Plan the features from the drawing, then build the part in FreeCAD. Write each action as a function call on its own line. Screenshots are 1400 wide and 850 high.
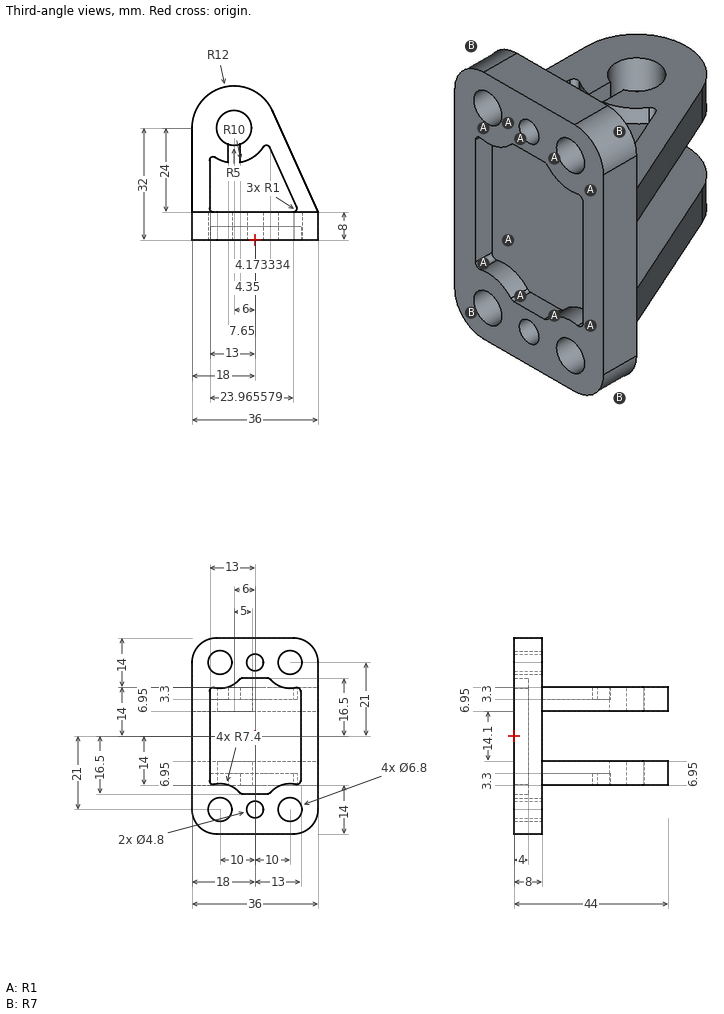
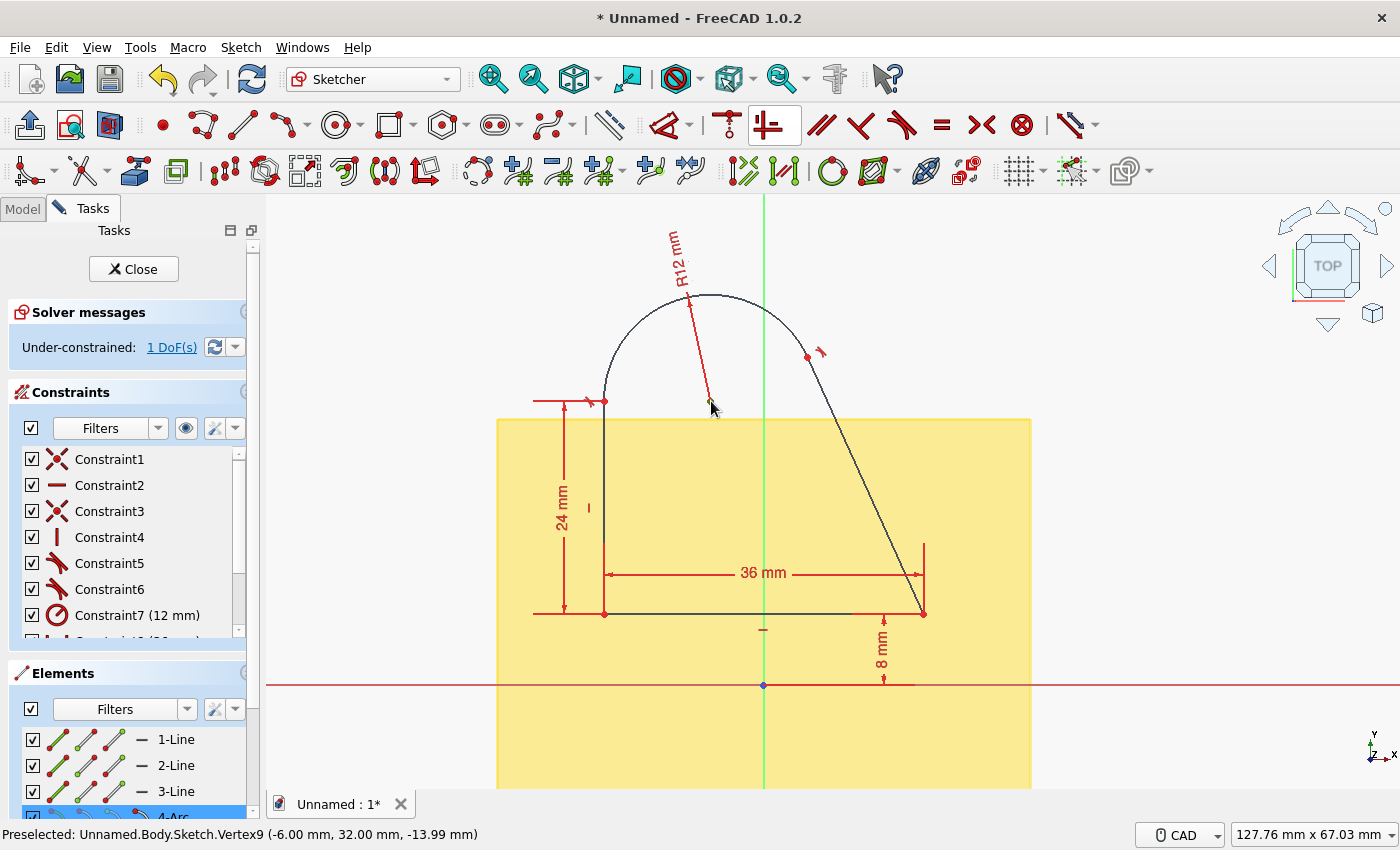
key(l)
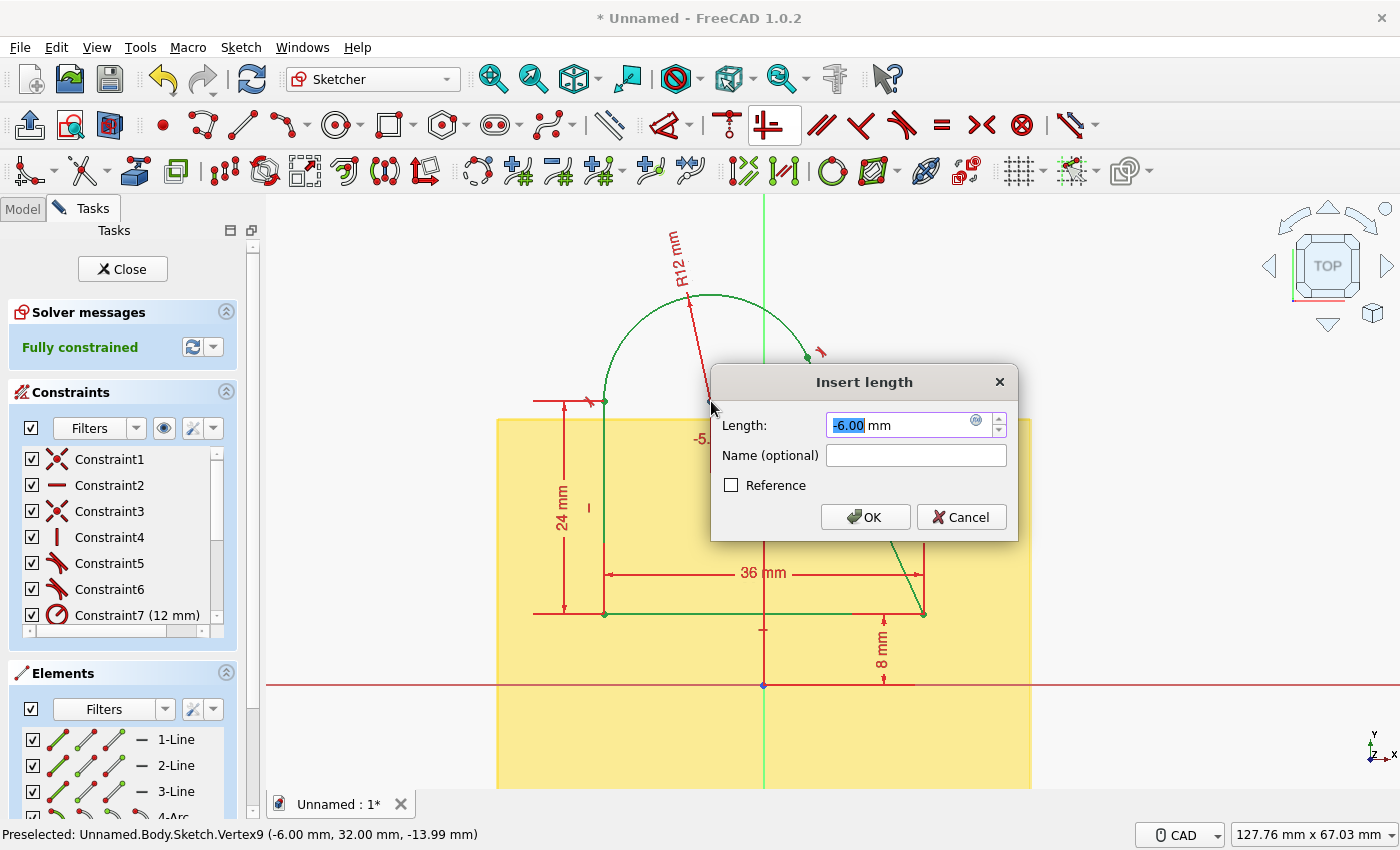
text(-6)
key(Return)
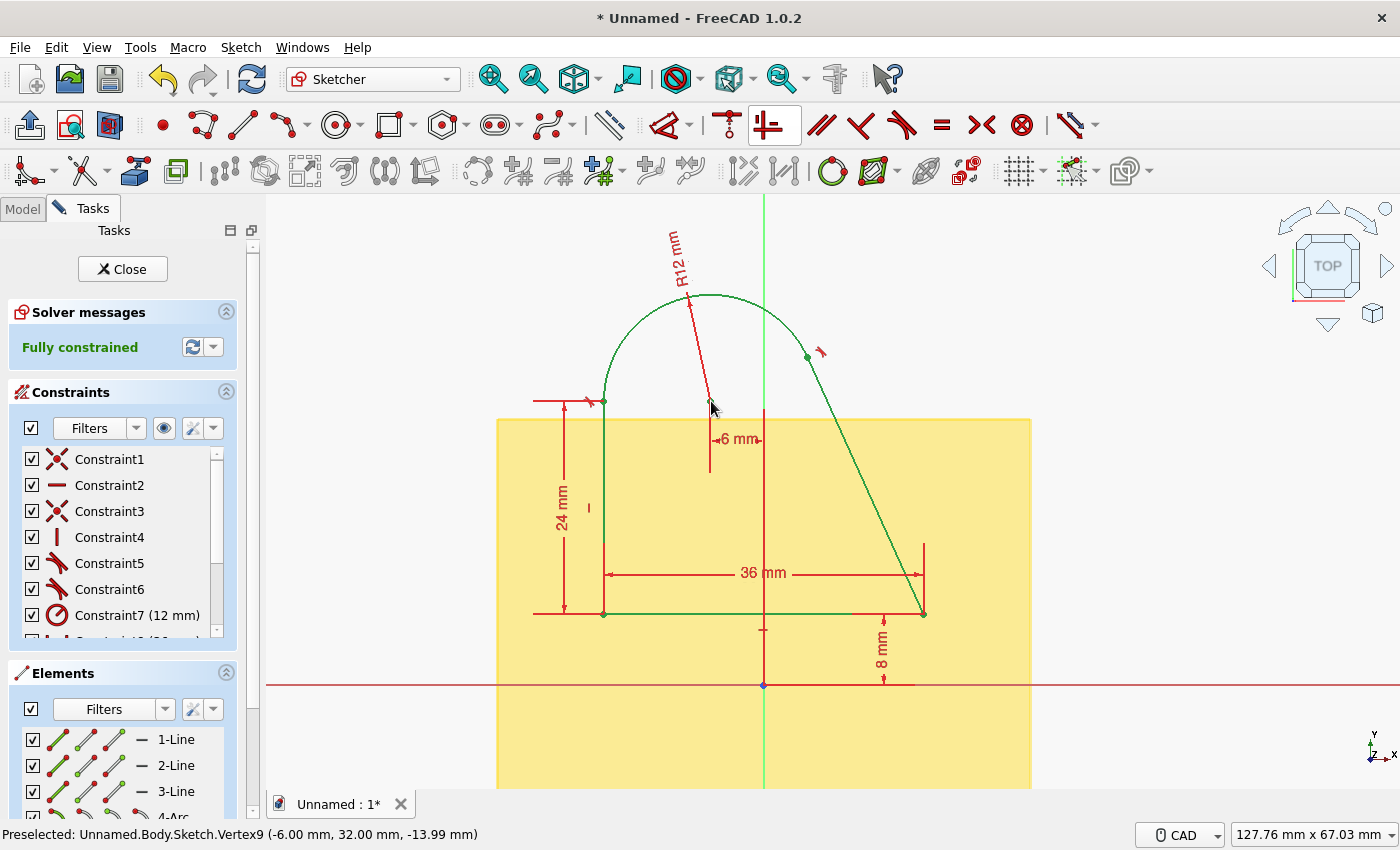
click(123, 269)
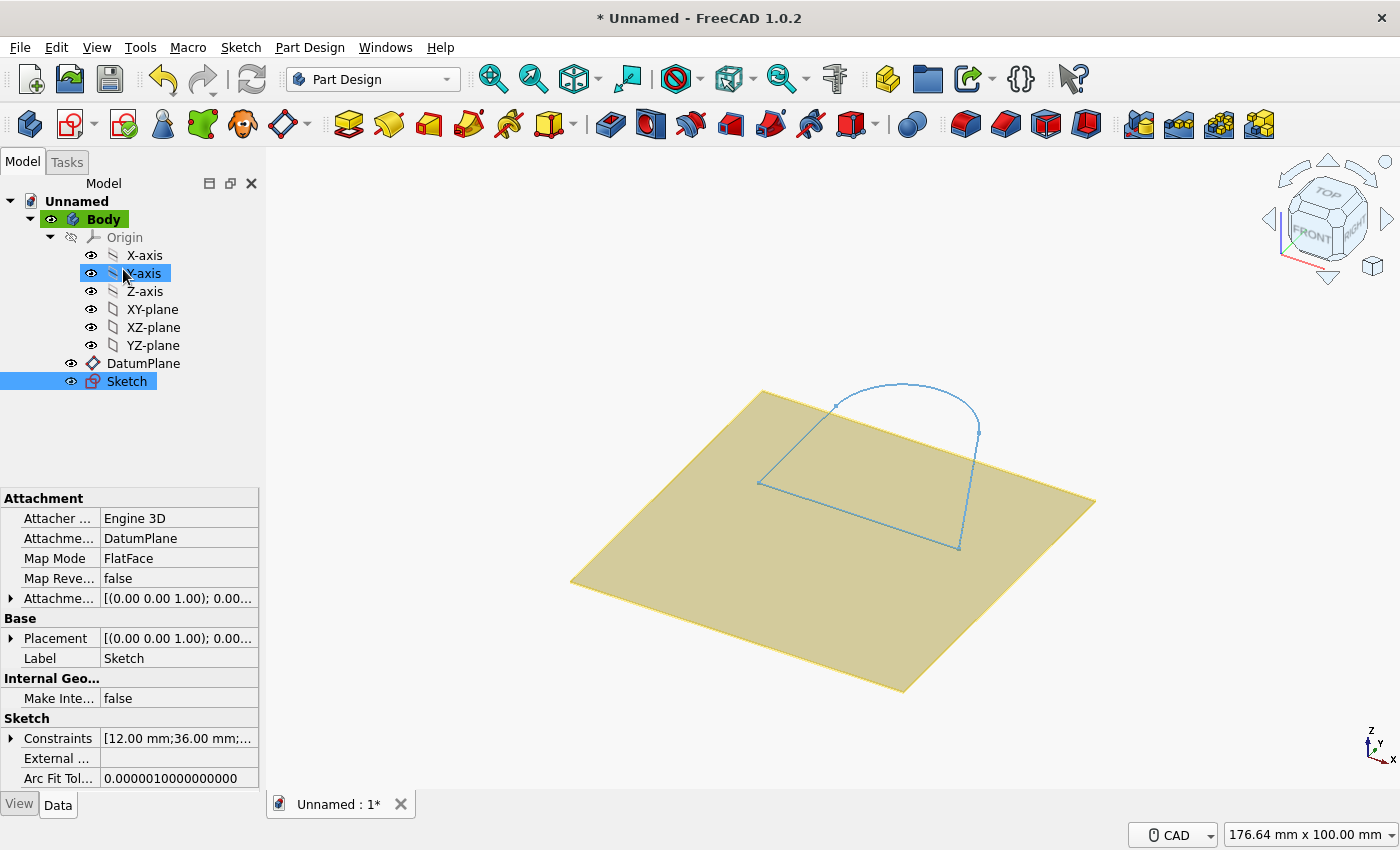
click(350, 124)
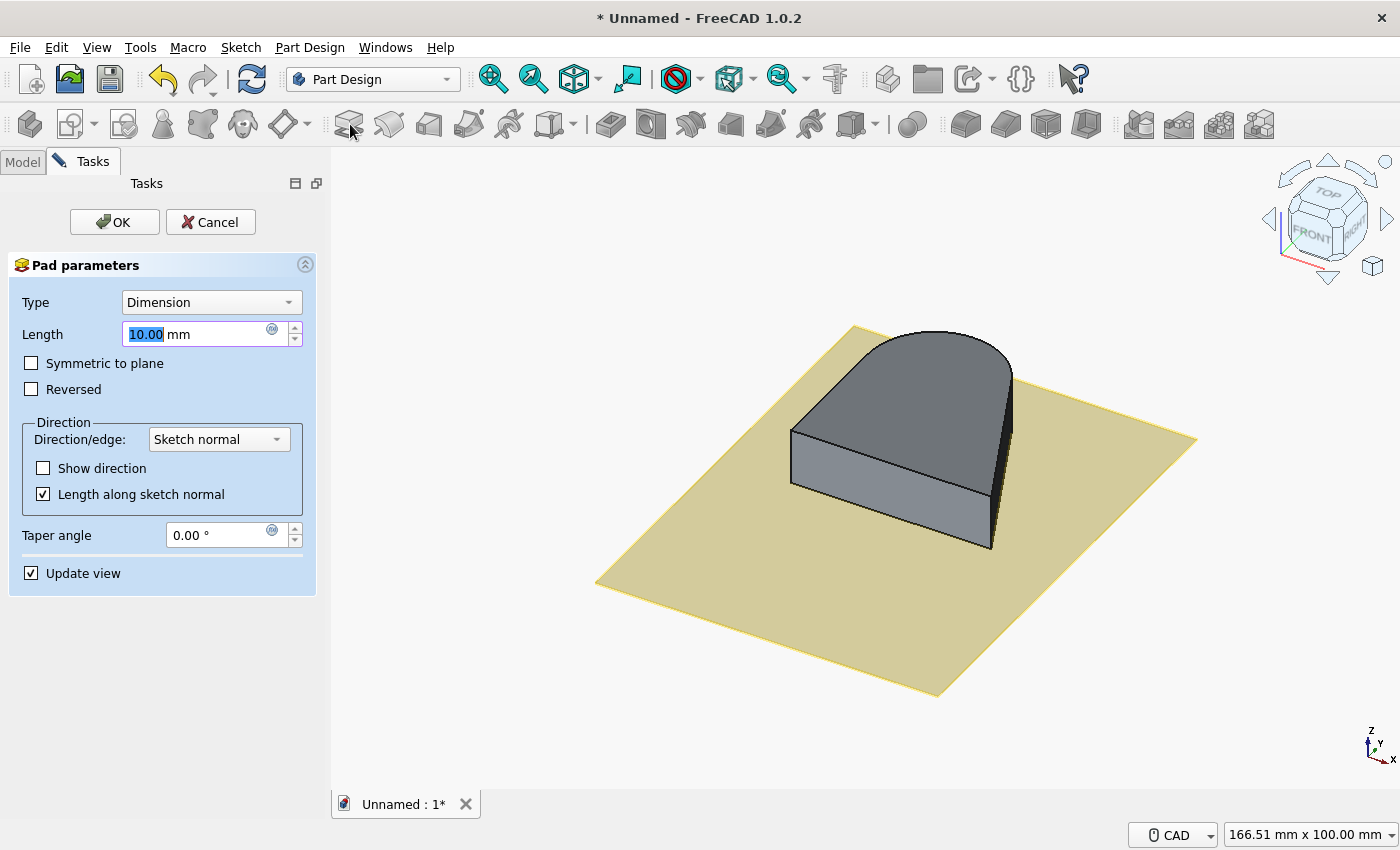
text(6.95)
key(Tab)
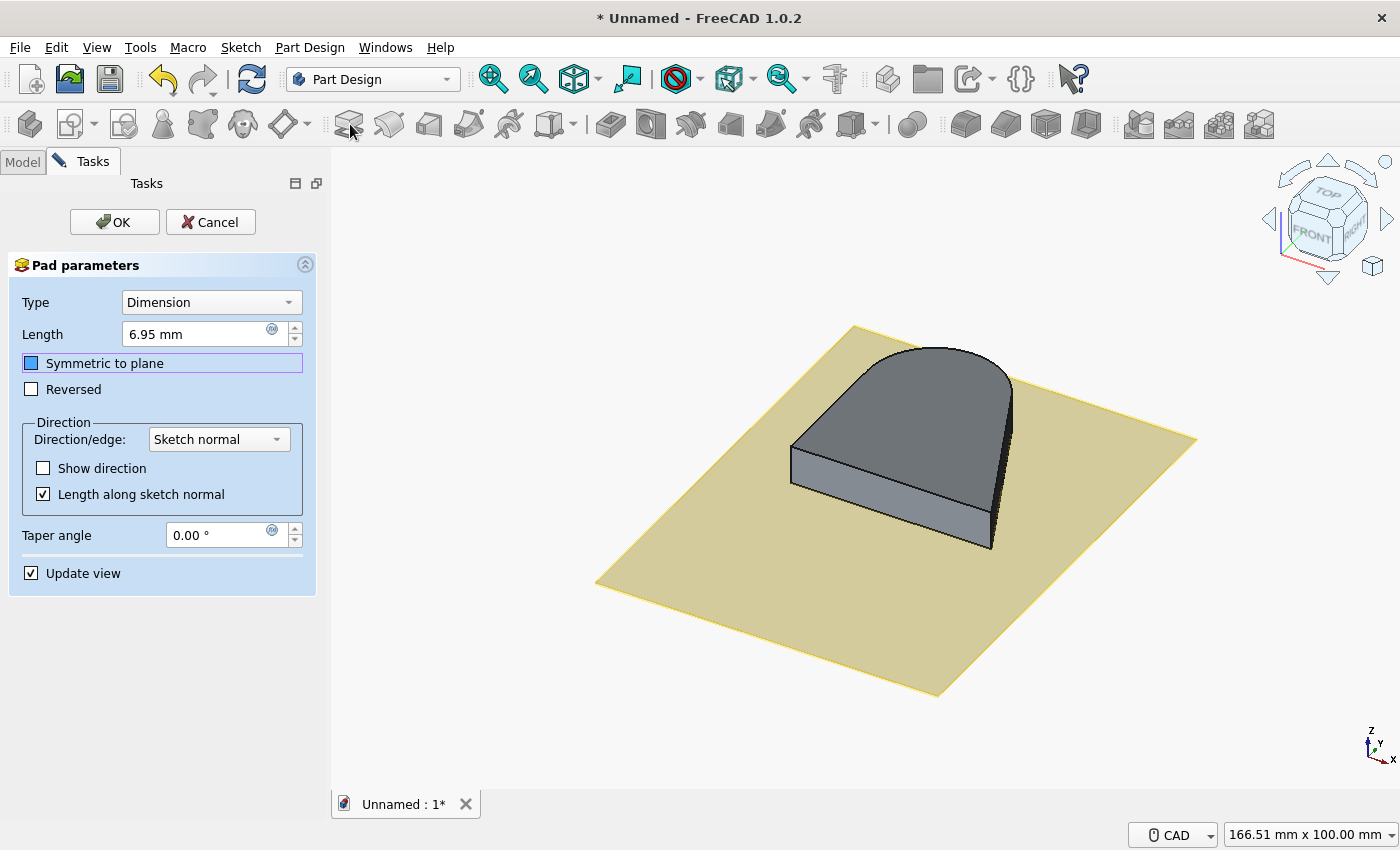
click(115, 222)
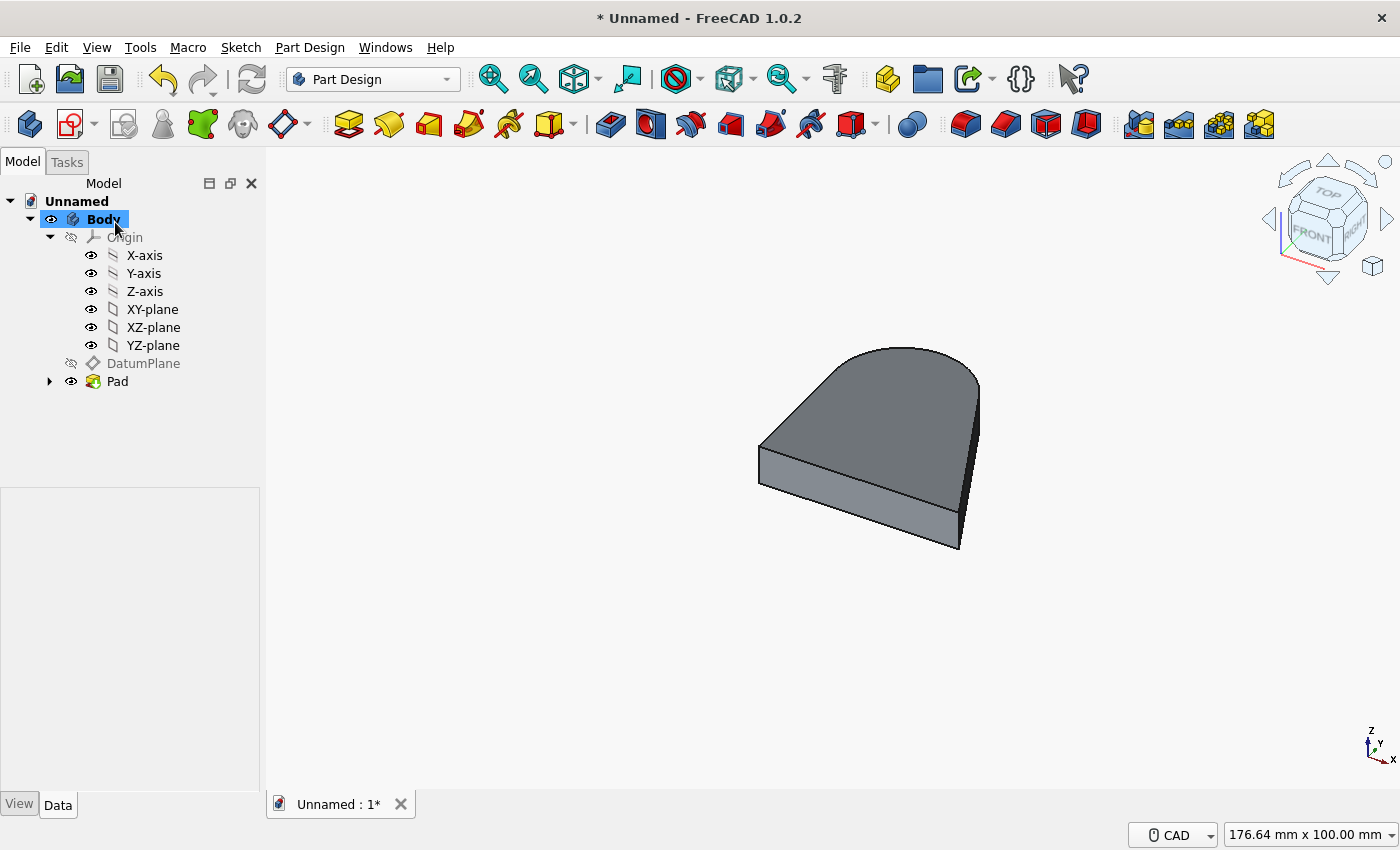
click(494, 80)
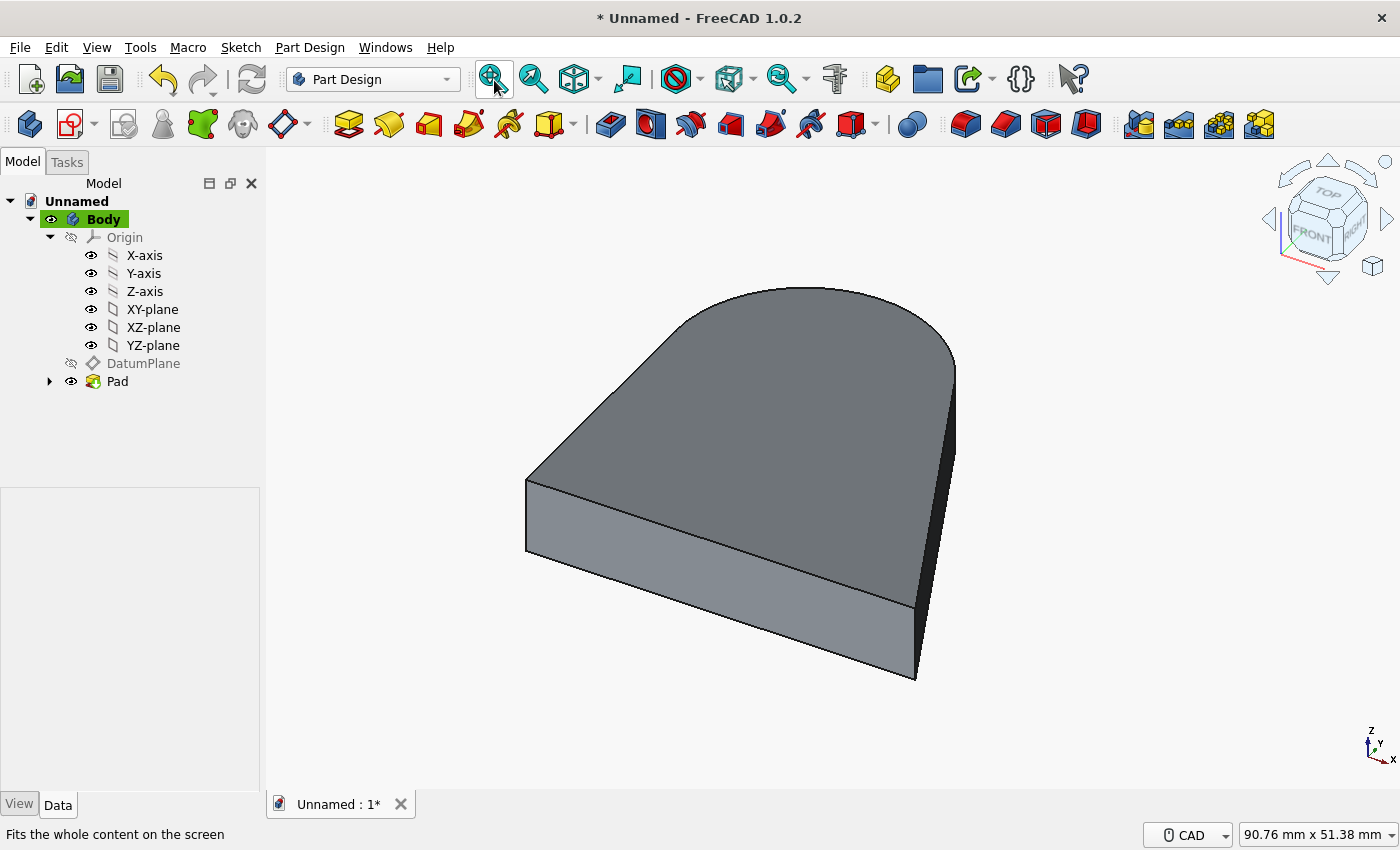
click(832, 616)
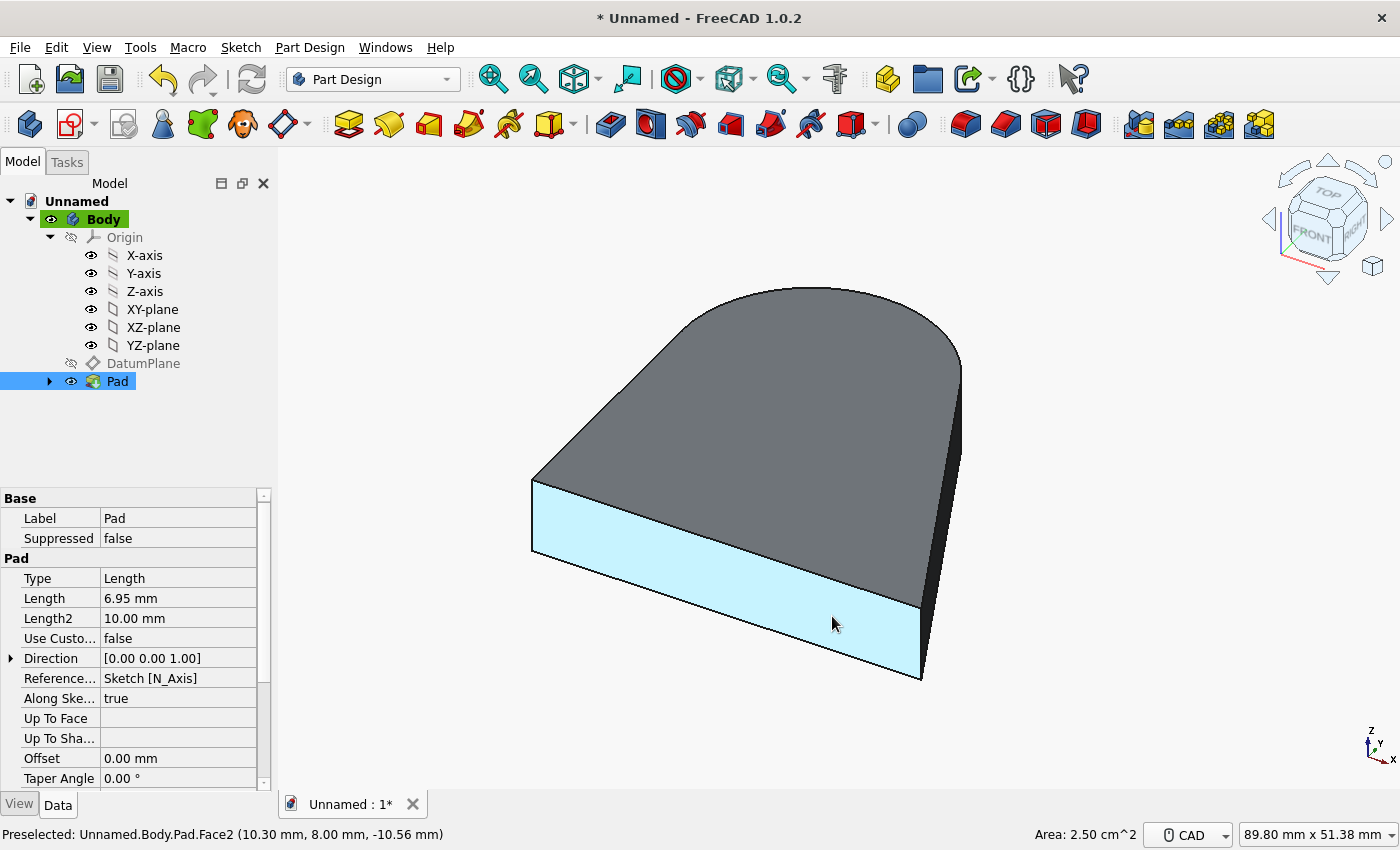
click(70, 124)